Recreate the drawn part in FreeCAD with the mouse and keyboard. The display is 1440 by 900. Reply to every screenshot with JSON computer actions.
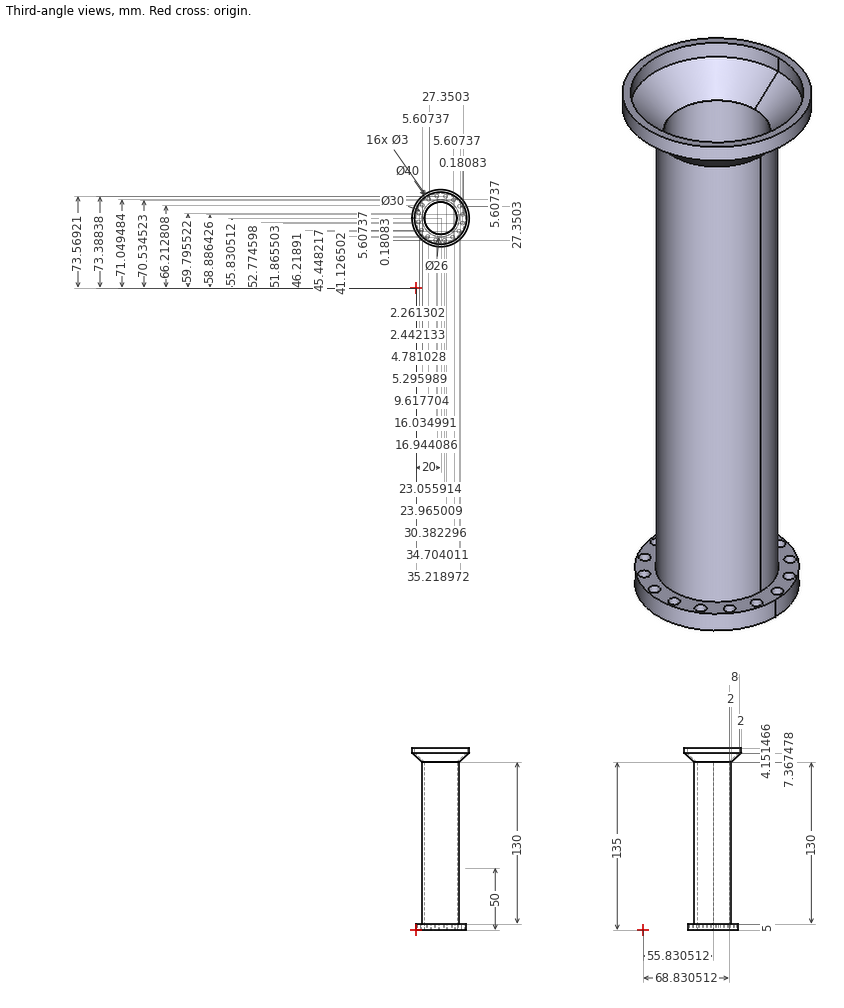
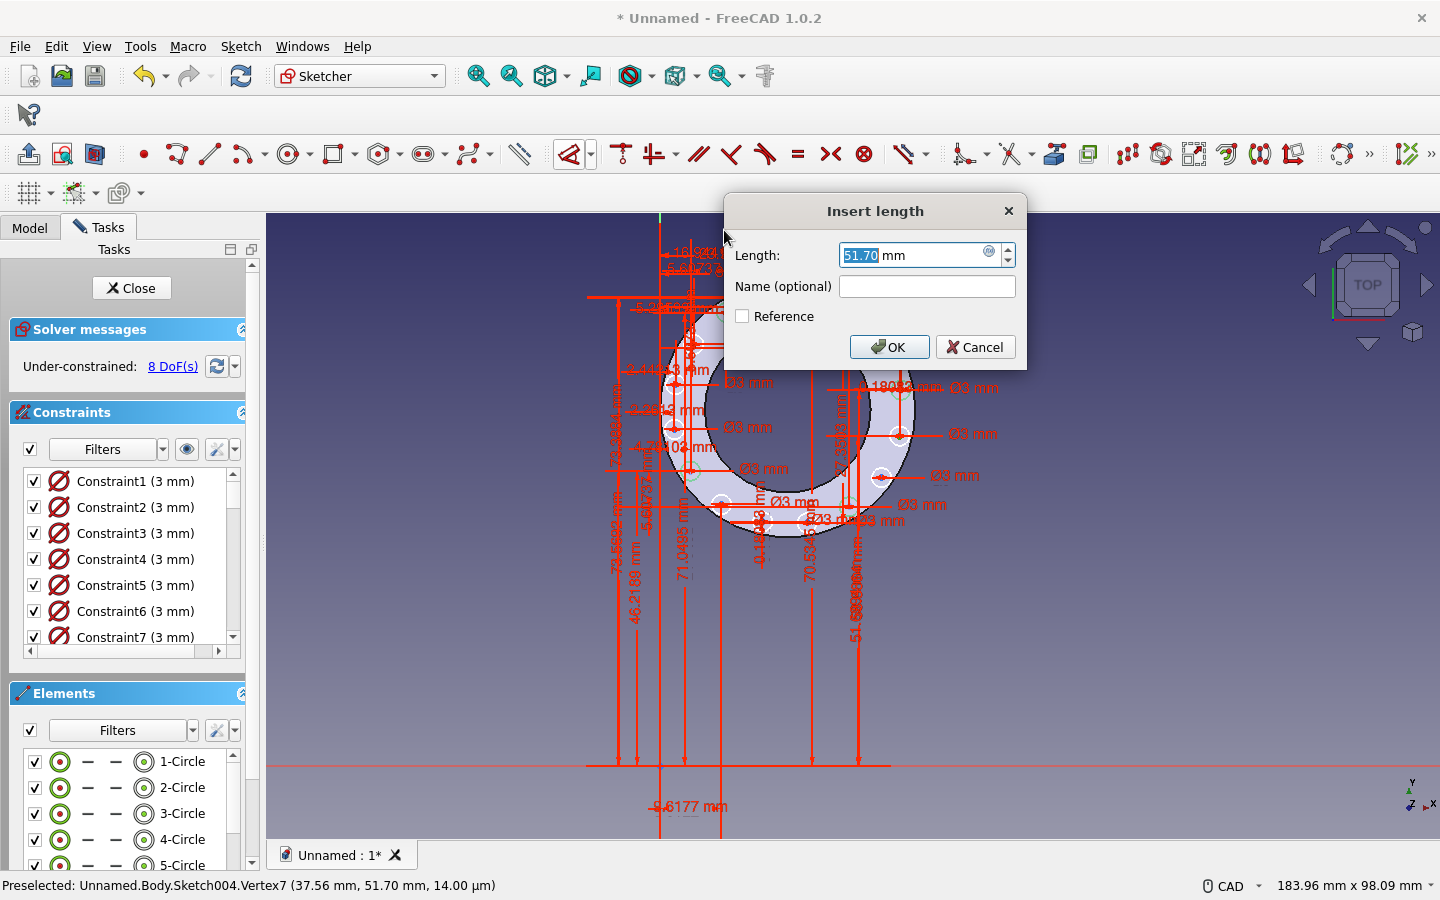
{"action": "type", "text": "51.865503"}
{"action": "key", "text": "Return"}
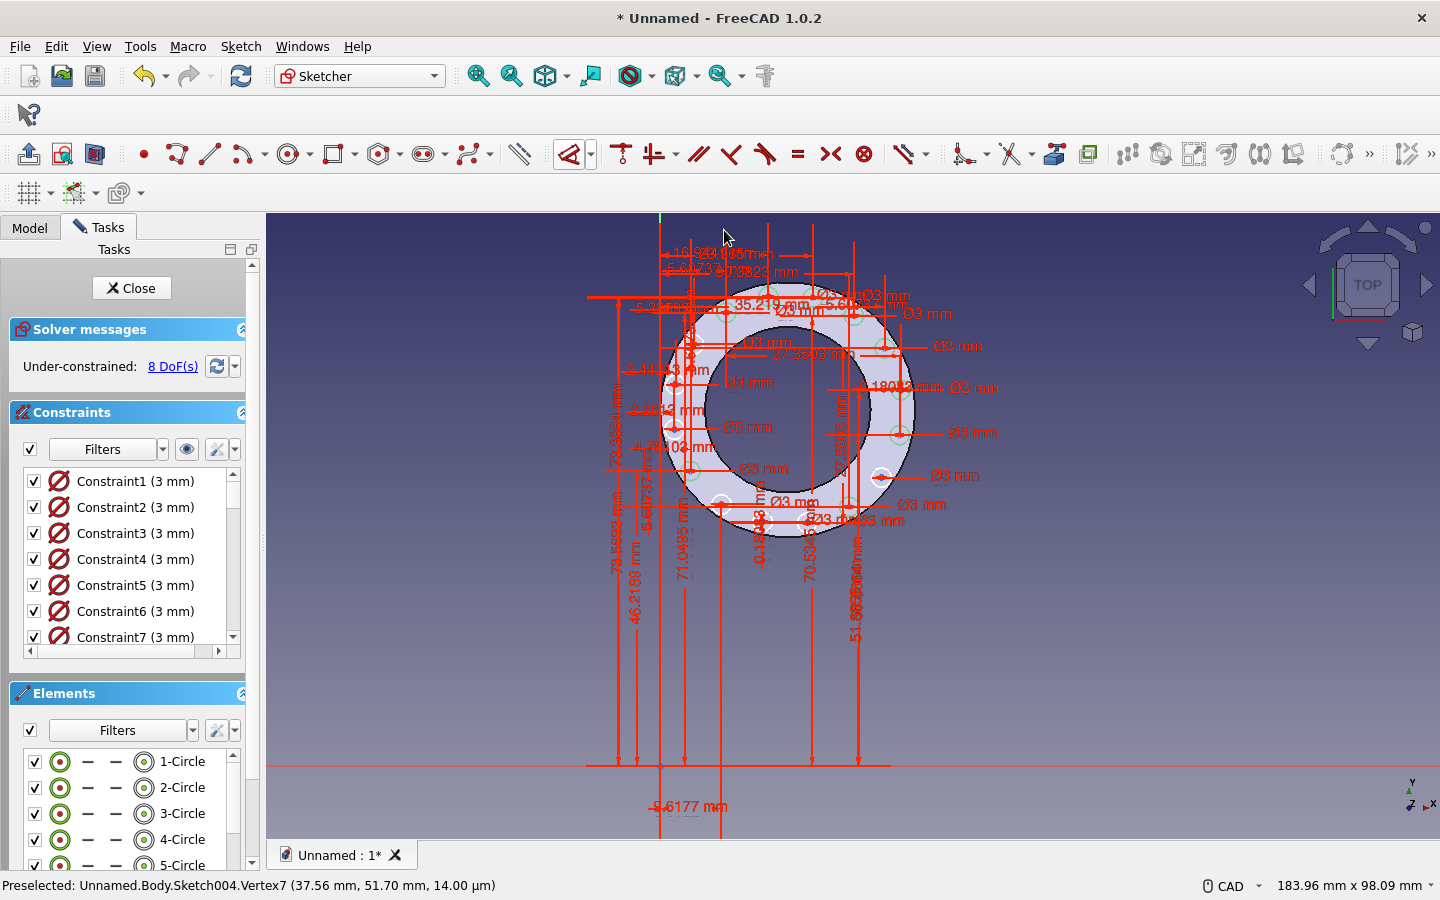
{"action": "left_click", "coordinate": [882, 478]}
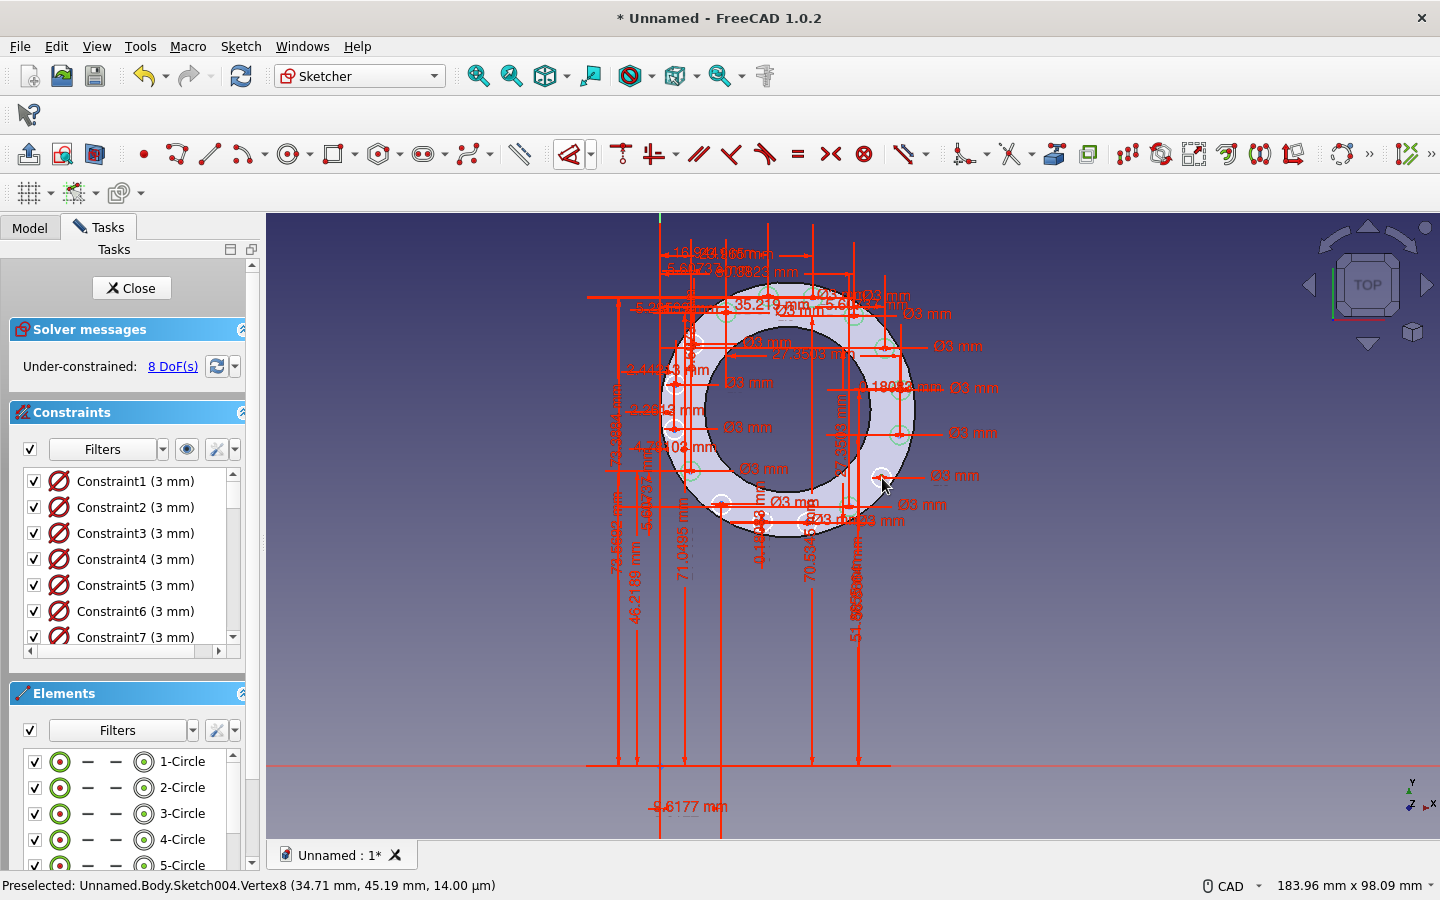
{"action": "key", "text": "l"}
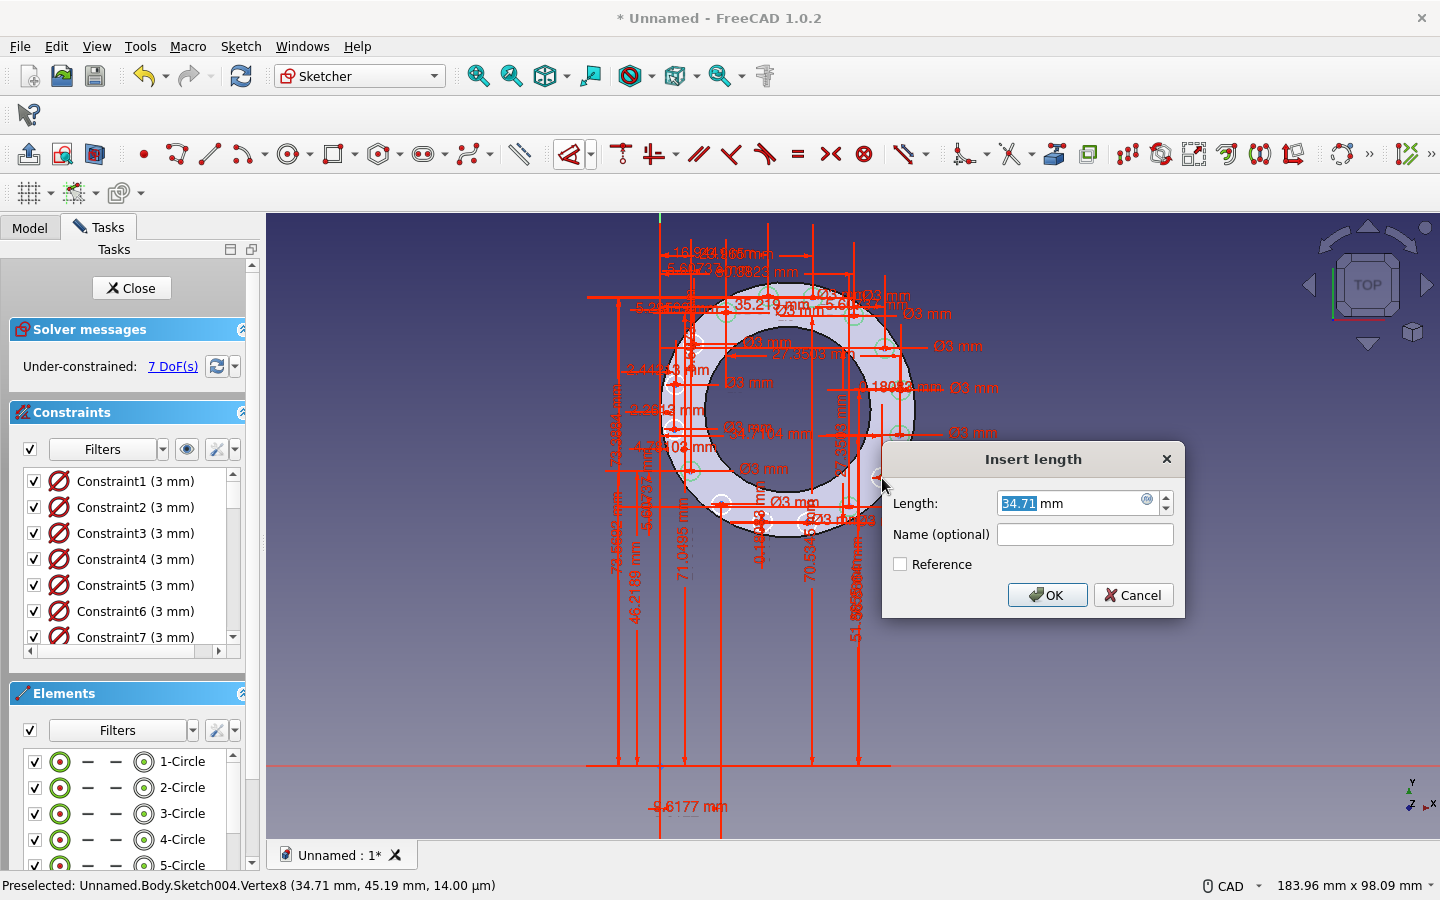
{"action": "type", "text": "34.704011"}
{"action": "key", "text": "Return"}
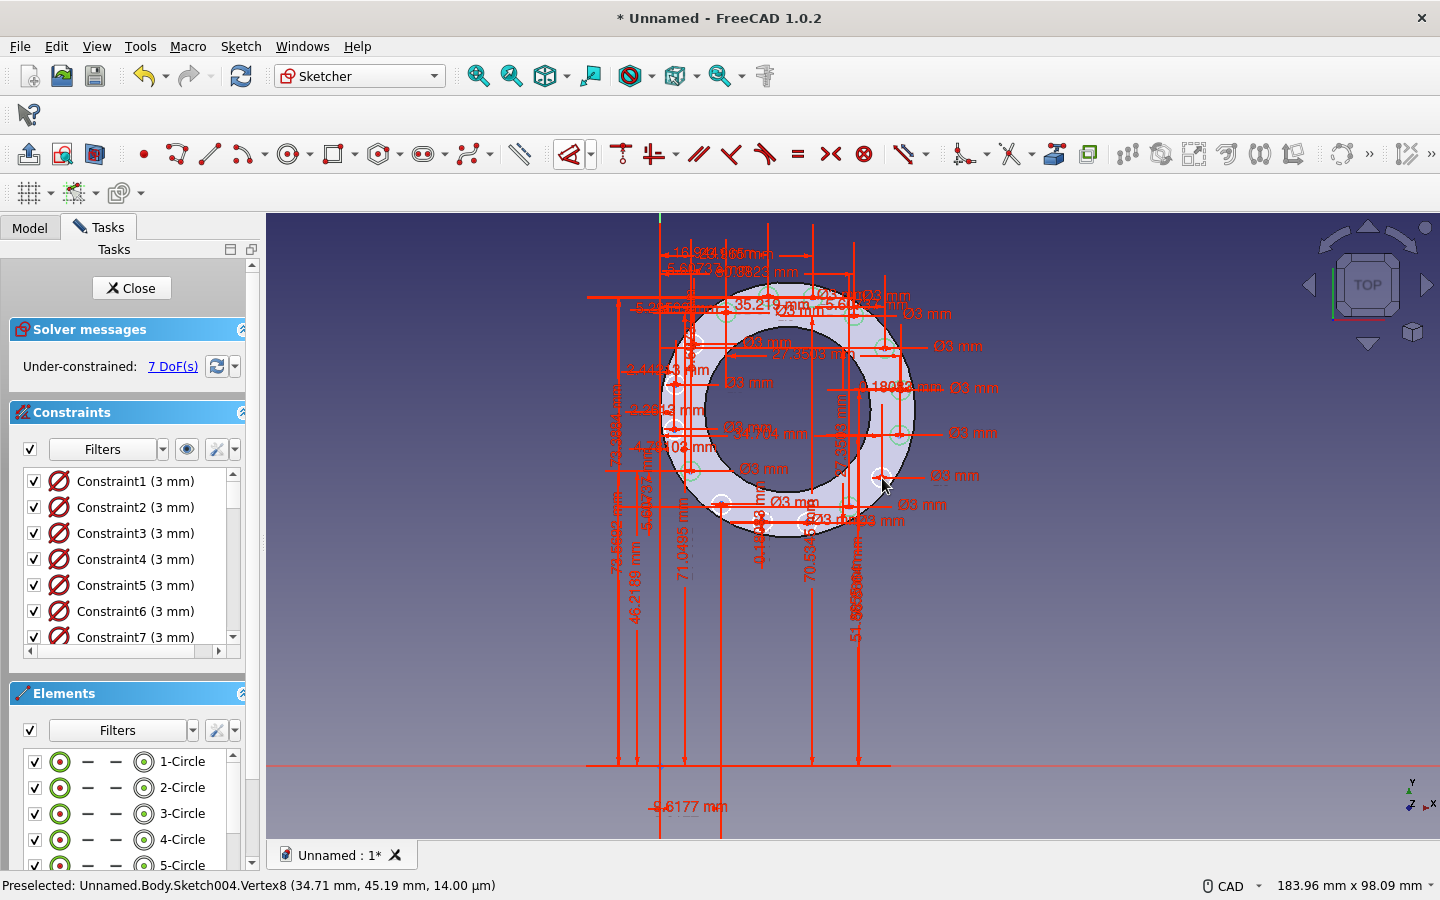
{"action": "left_click", "coordinate": [882, 478]}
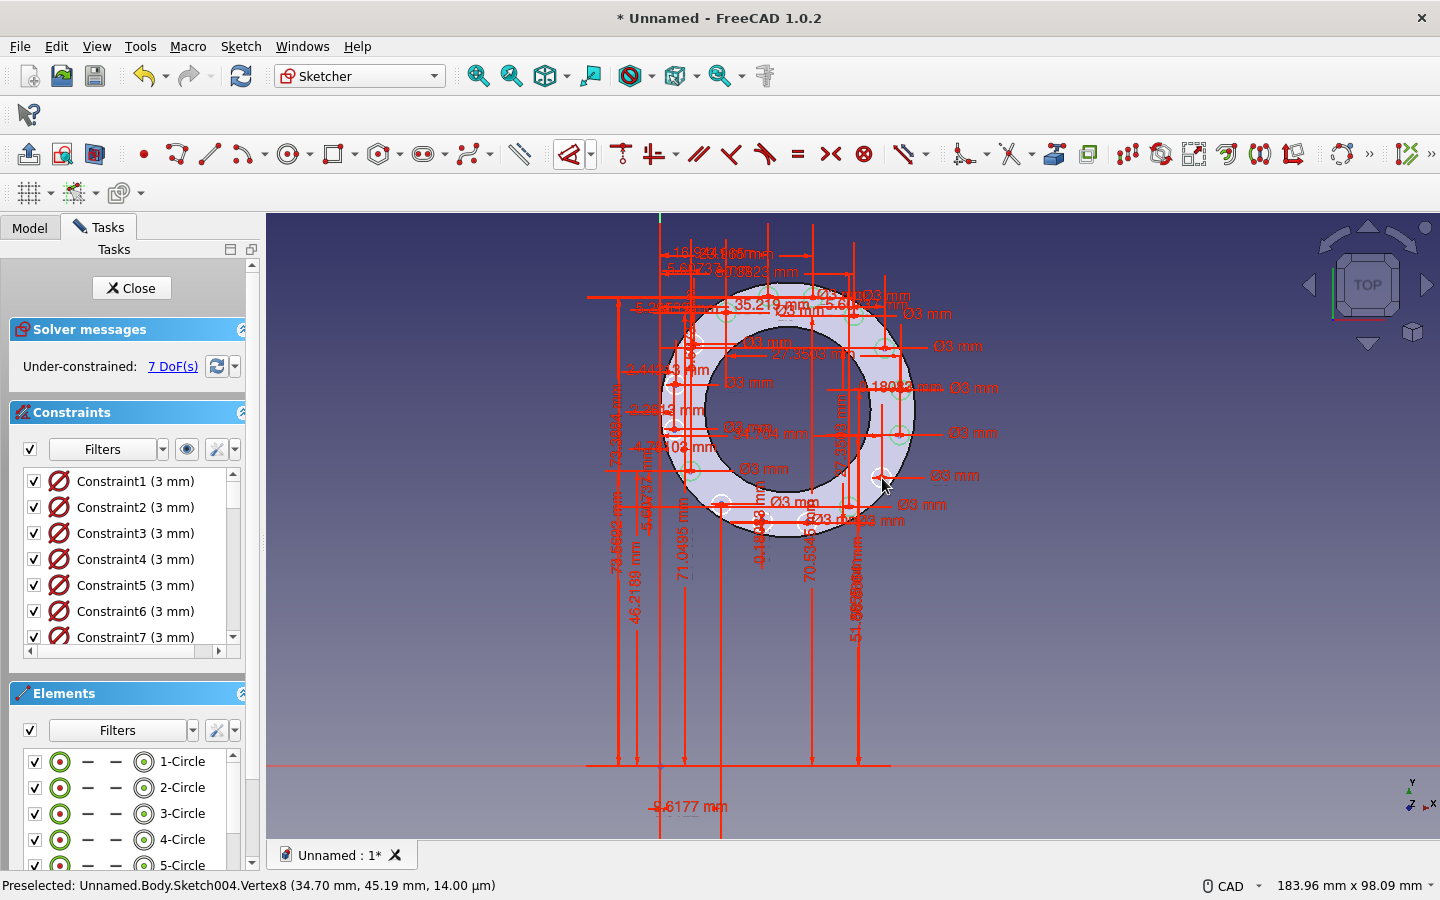
{"action": "key", "text": "i"}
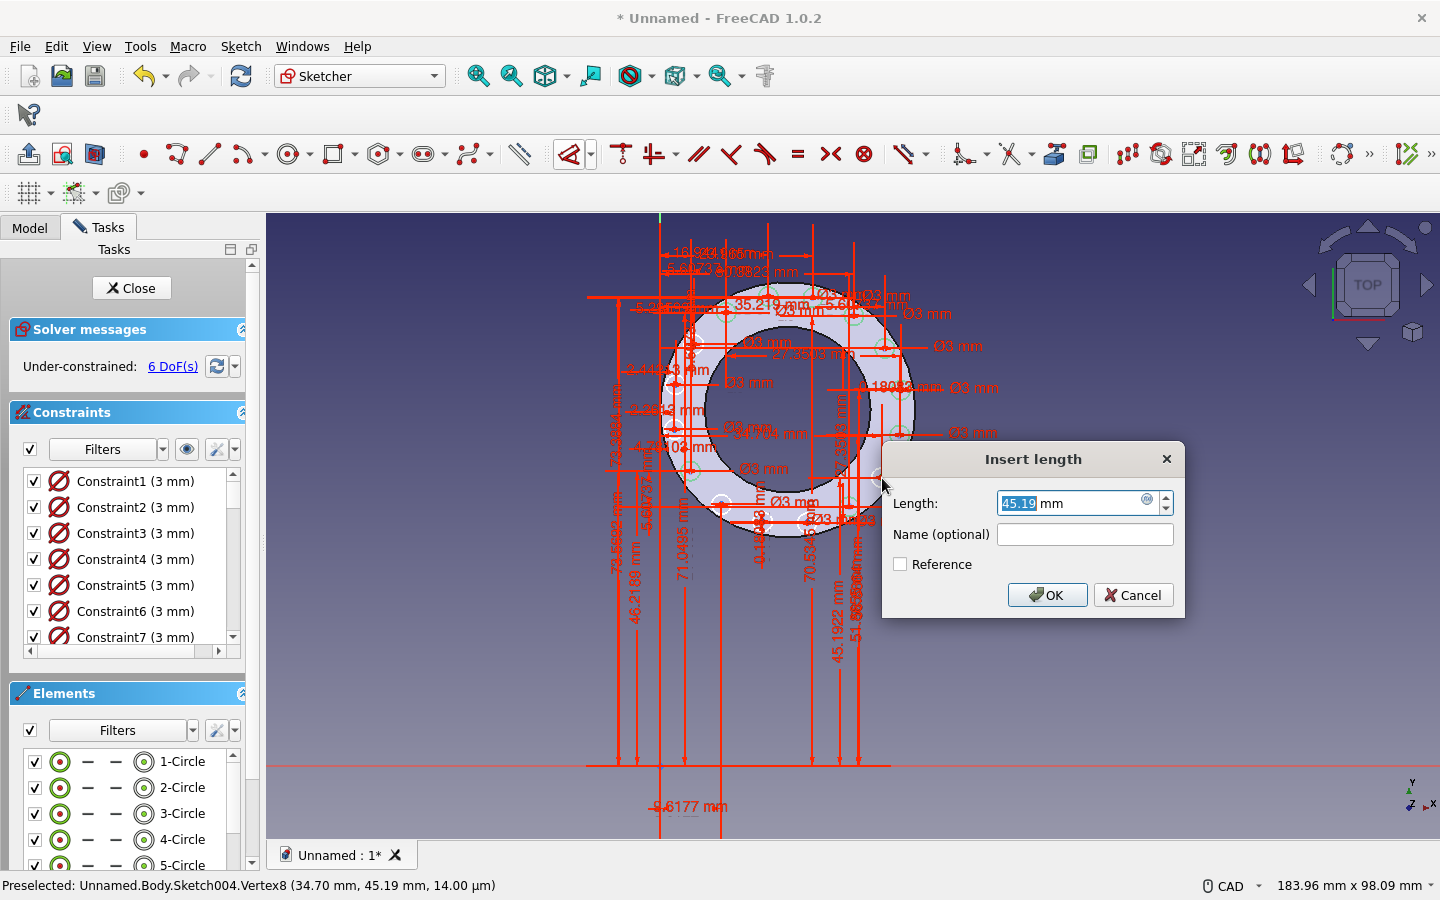
{"action": "type", "text": "45.448217"}
{"action": "key", "text": "Return"}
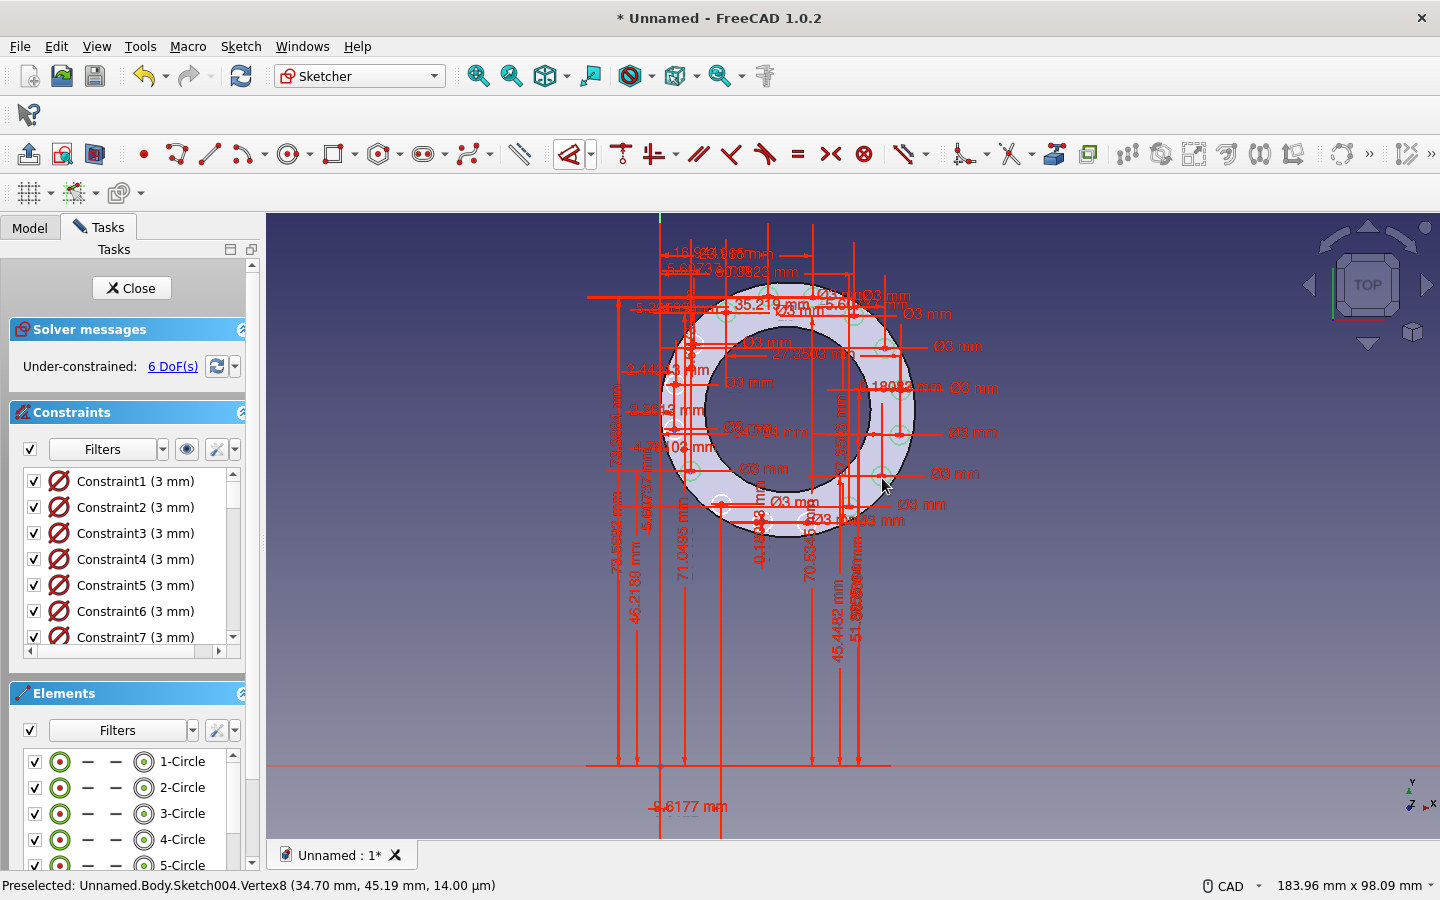
{"action": "left_click", "coordinate": [807, 523]}